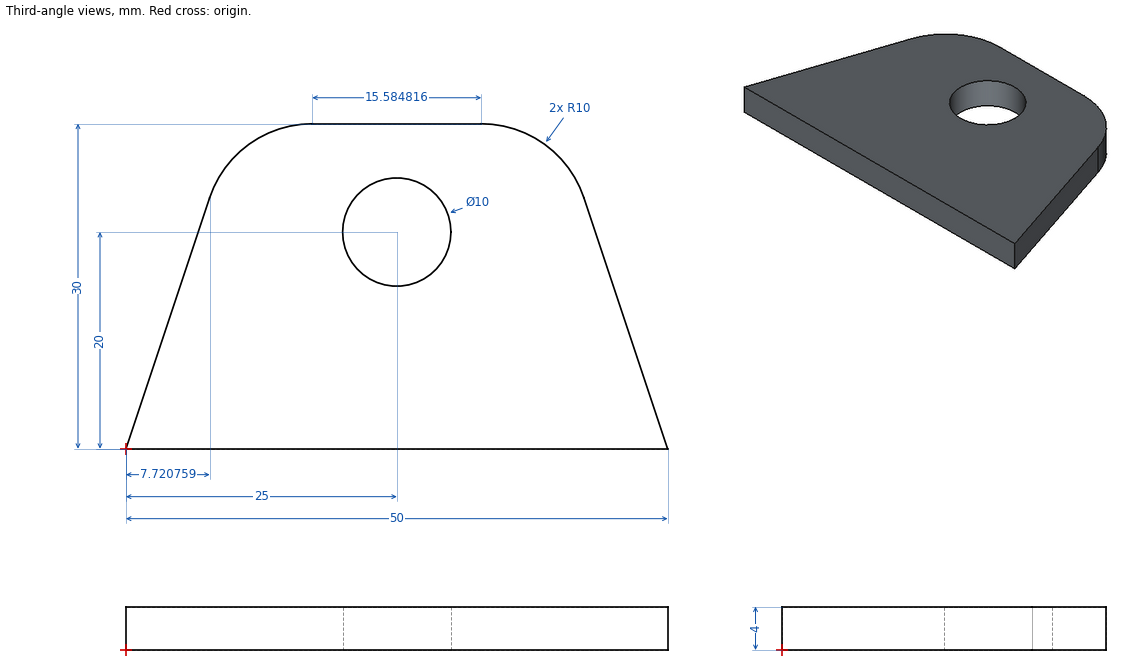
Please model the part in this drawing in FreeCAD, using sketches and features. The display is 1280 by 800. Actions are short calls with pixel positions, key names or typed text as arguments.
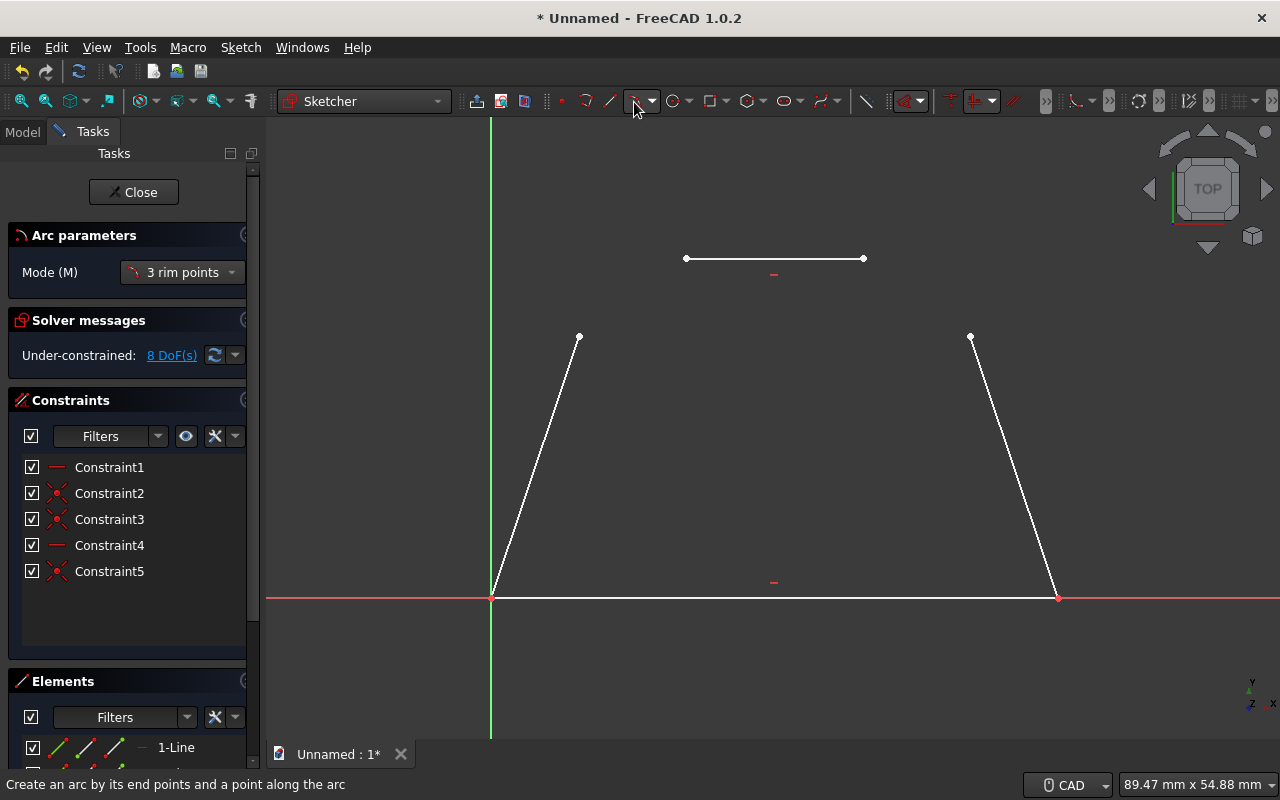
click(686, 259)
click(579, 337)
click(620, 279)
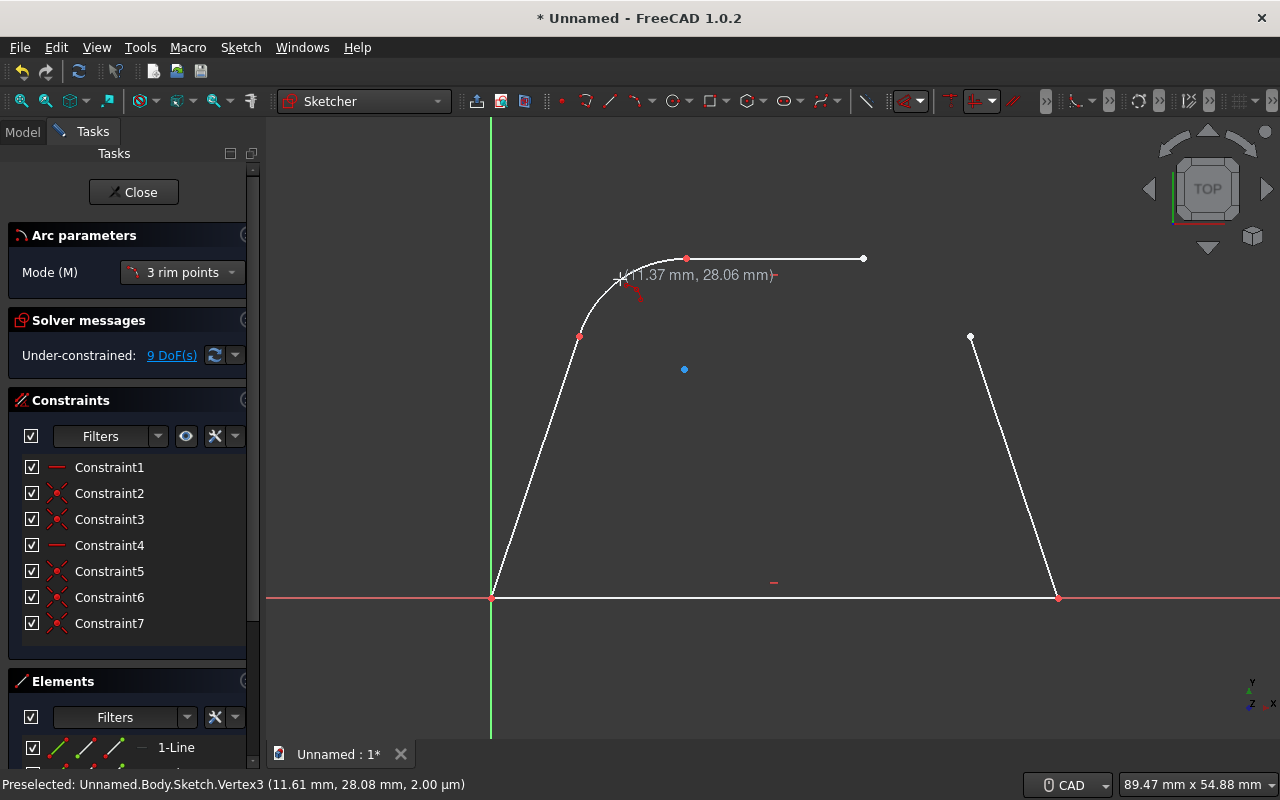
click(970, 337)
click(863, 259)
click(929, 279)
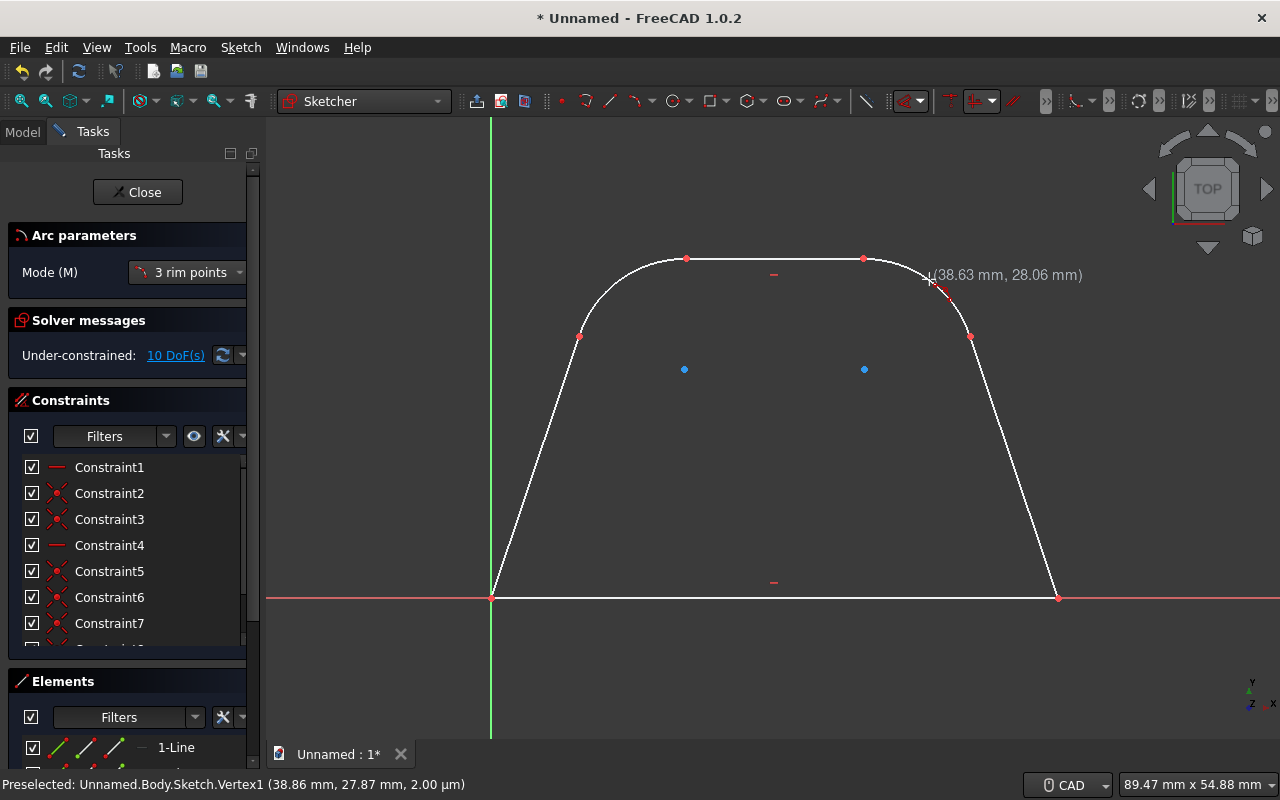
click(674, 102)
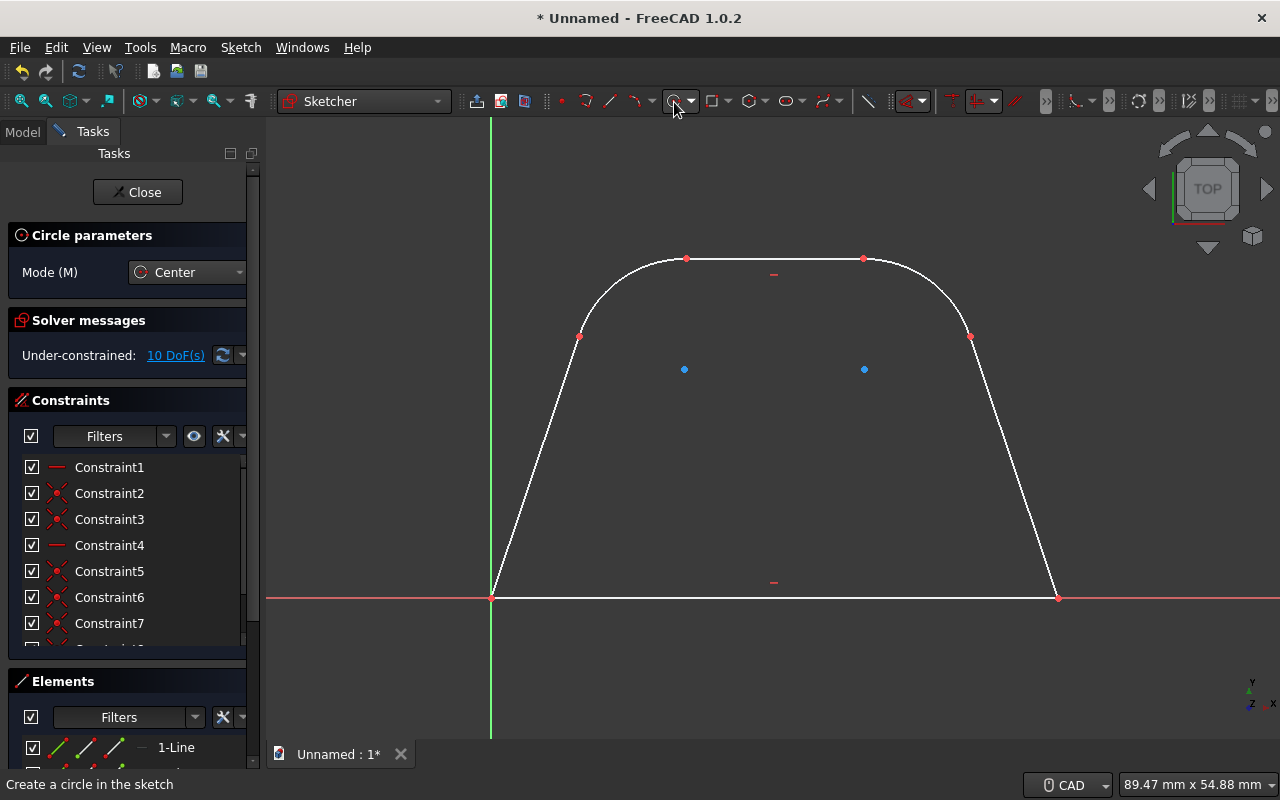
click(774, 371)
click(815, 331)
key(Escape)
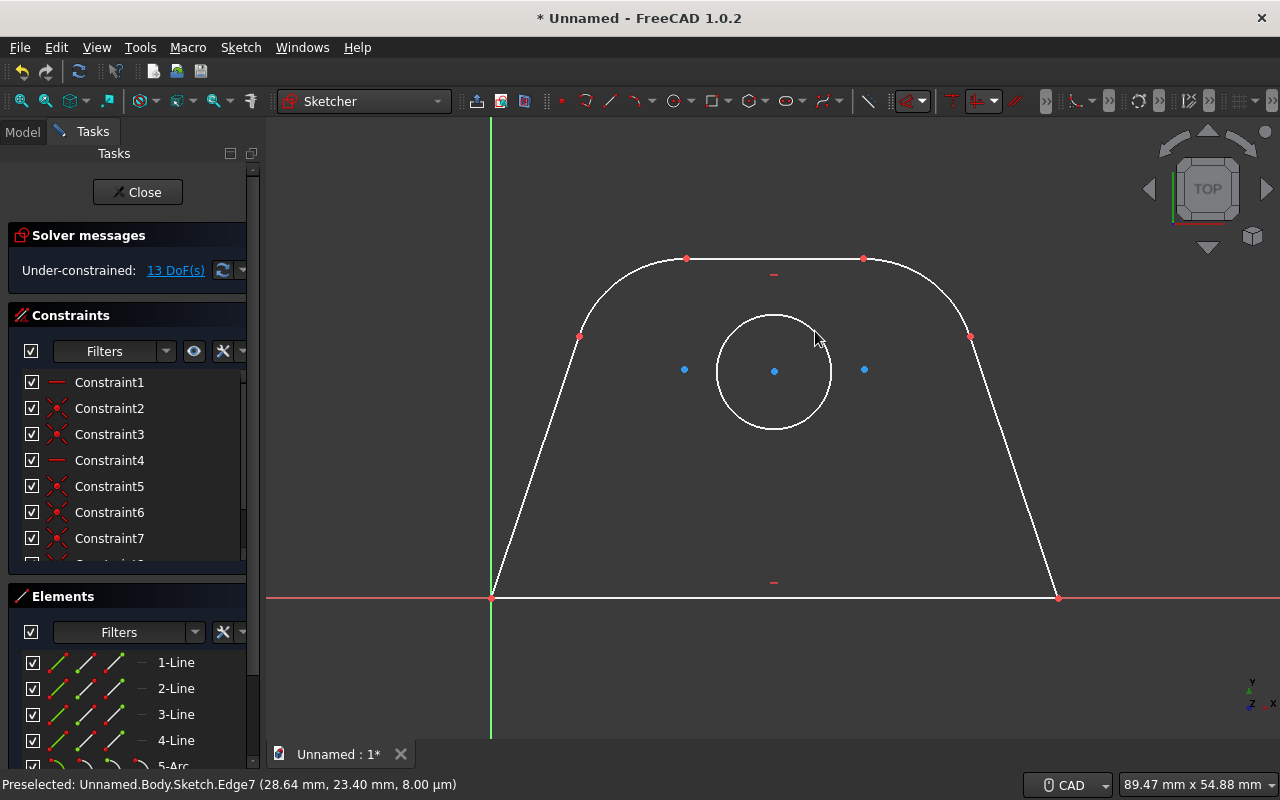
click(810, 259)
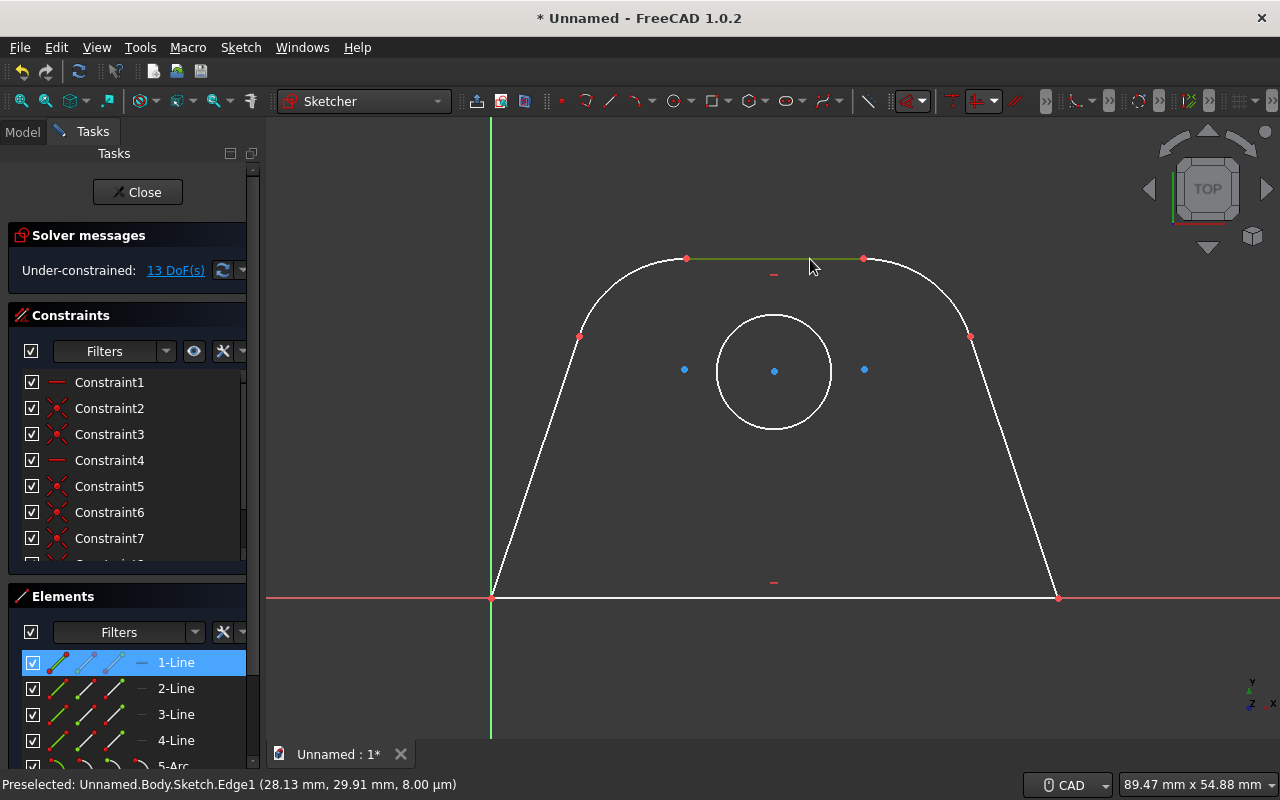
click(644, 267)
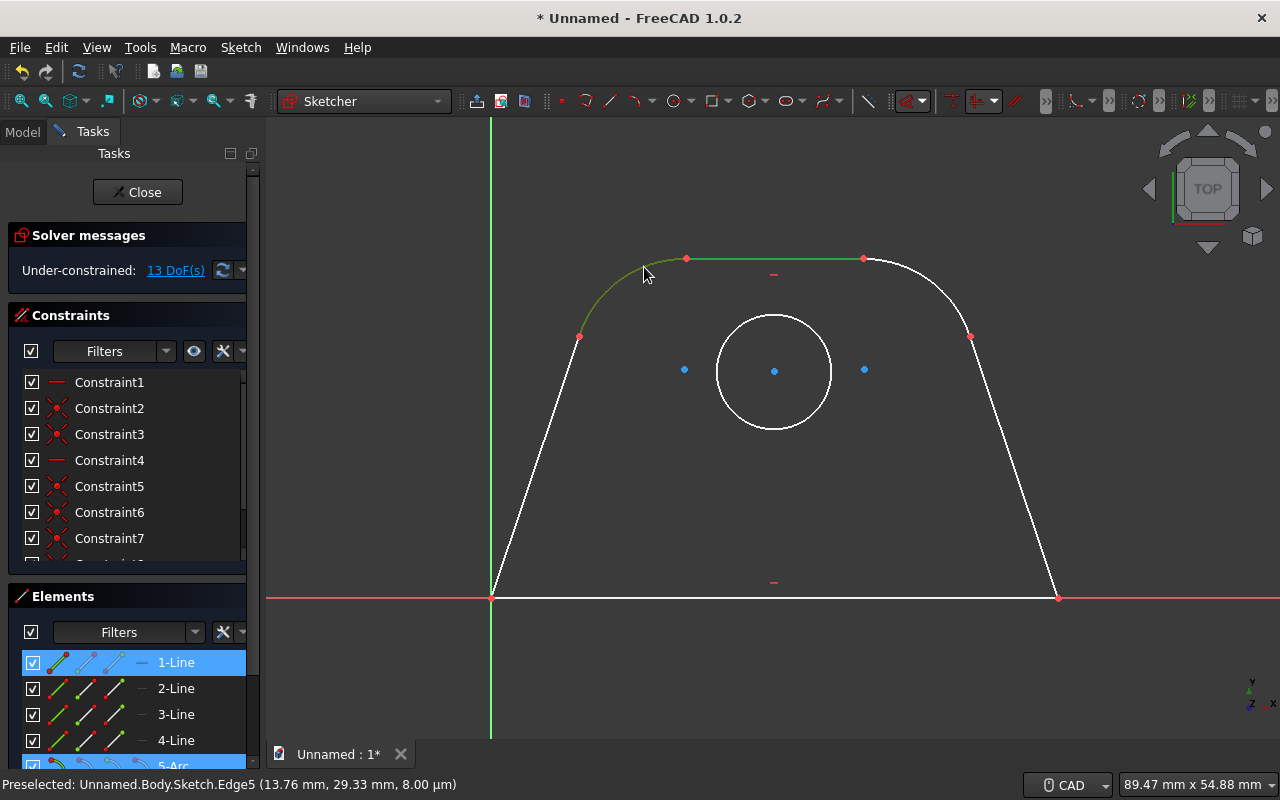
key(t)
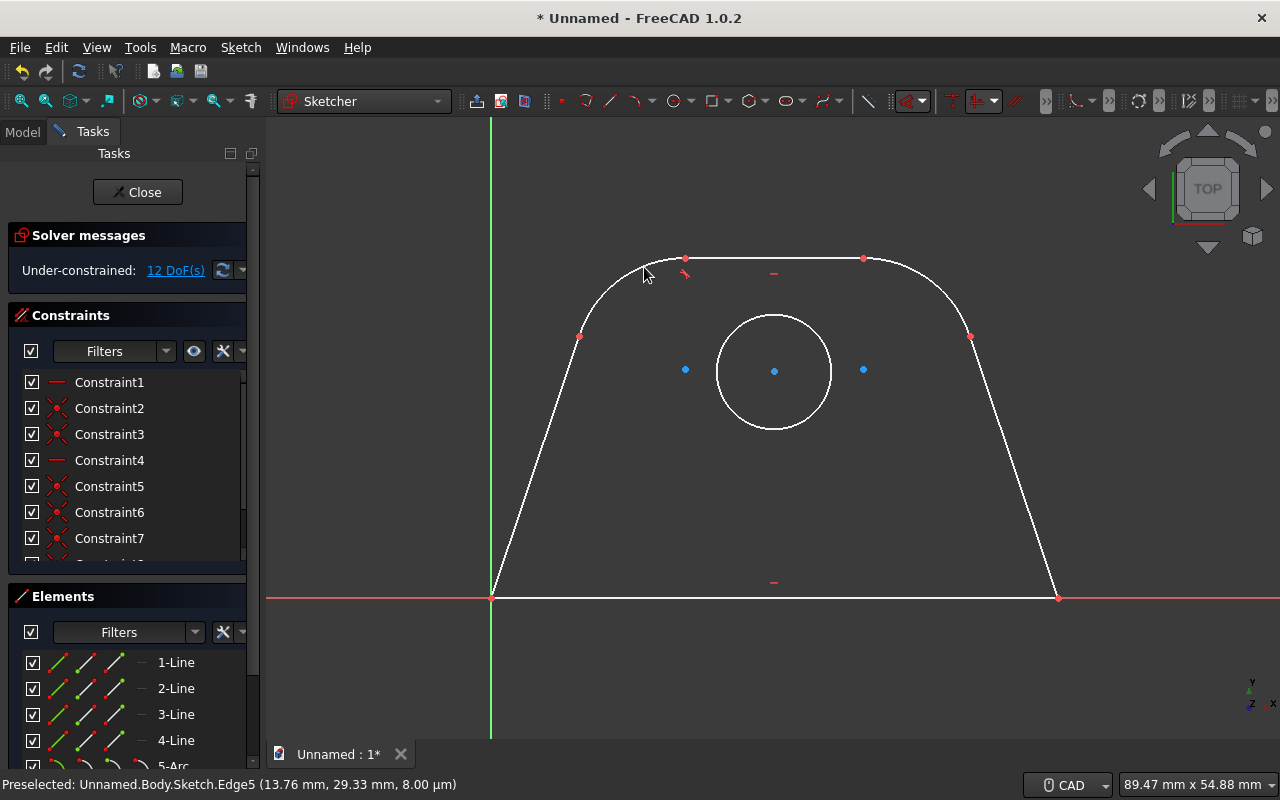
click(810, 258)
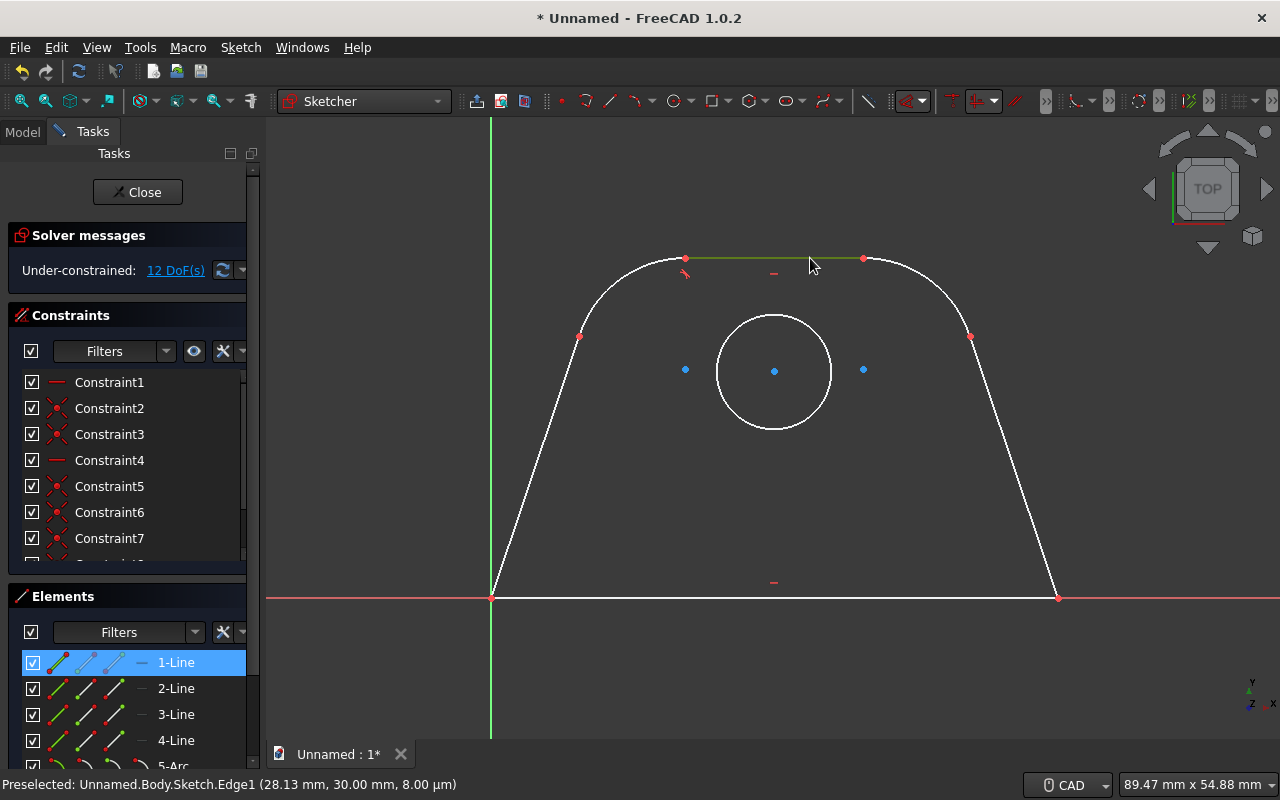
click(950, 300)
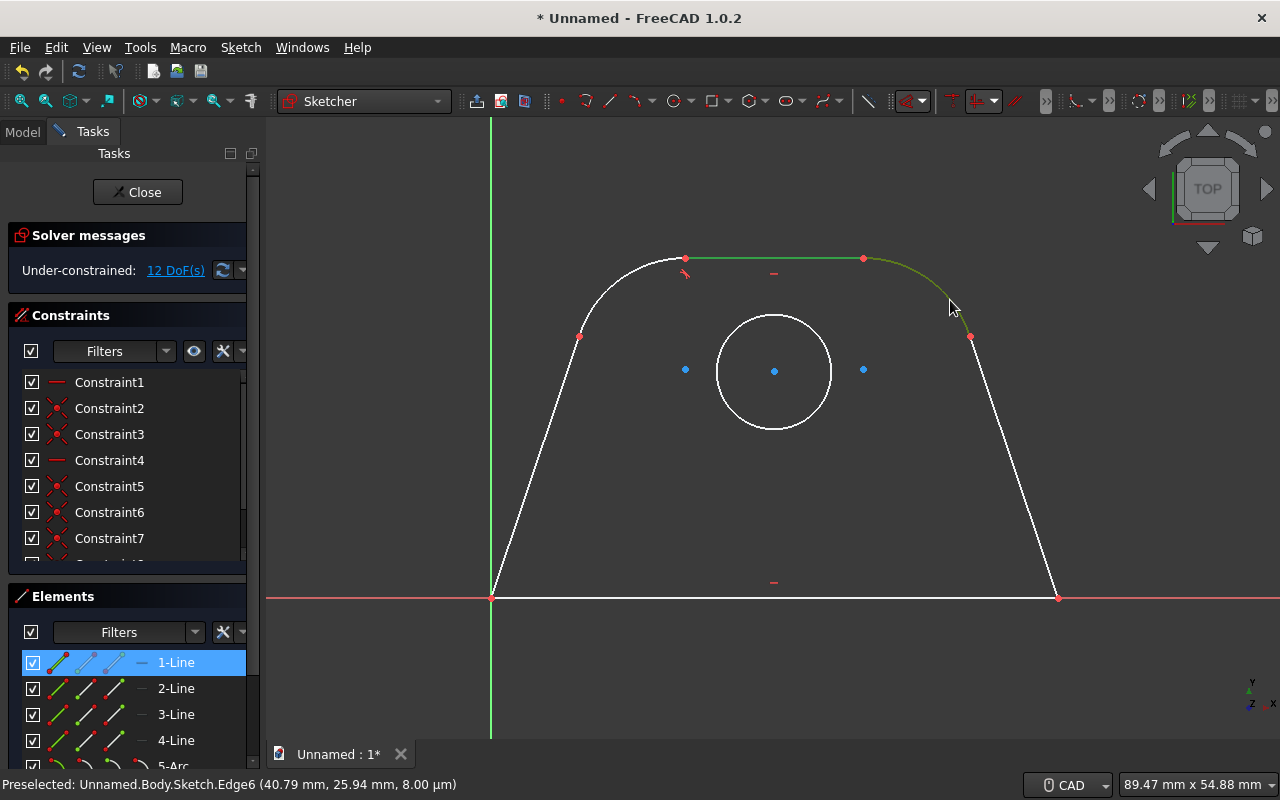
key(t)